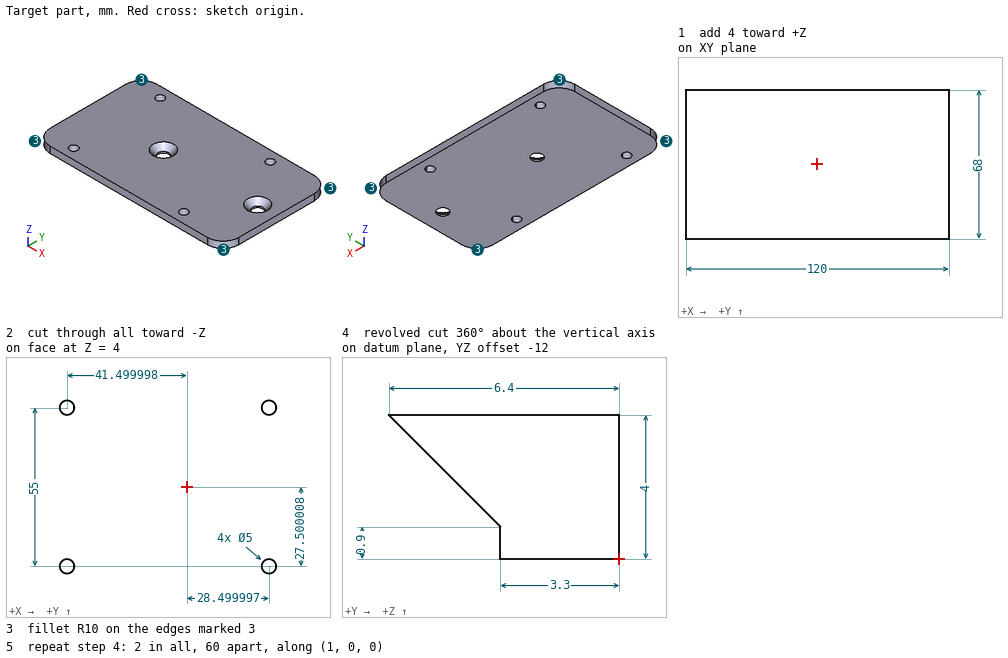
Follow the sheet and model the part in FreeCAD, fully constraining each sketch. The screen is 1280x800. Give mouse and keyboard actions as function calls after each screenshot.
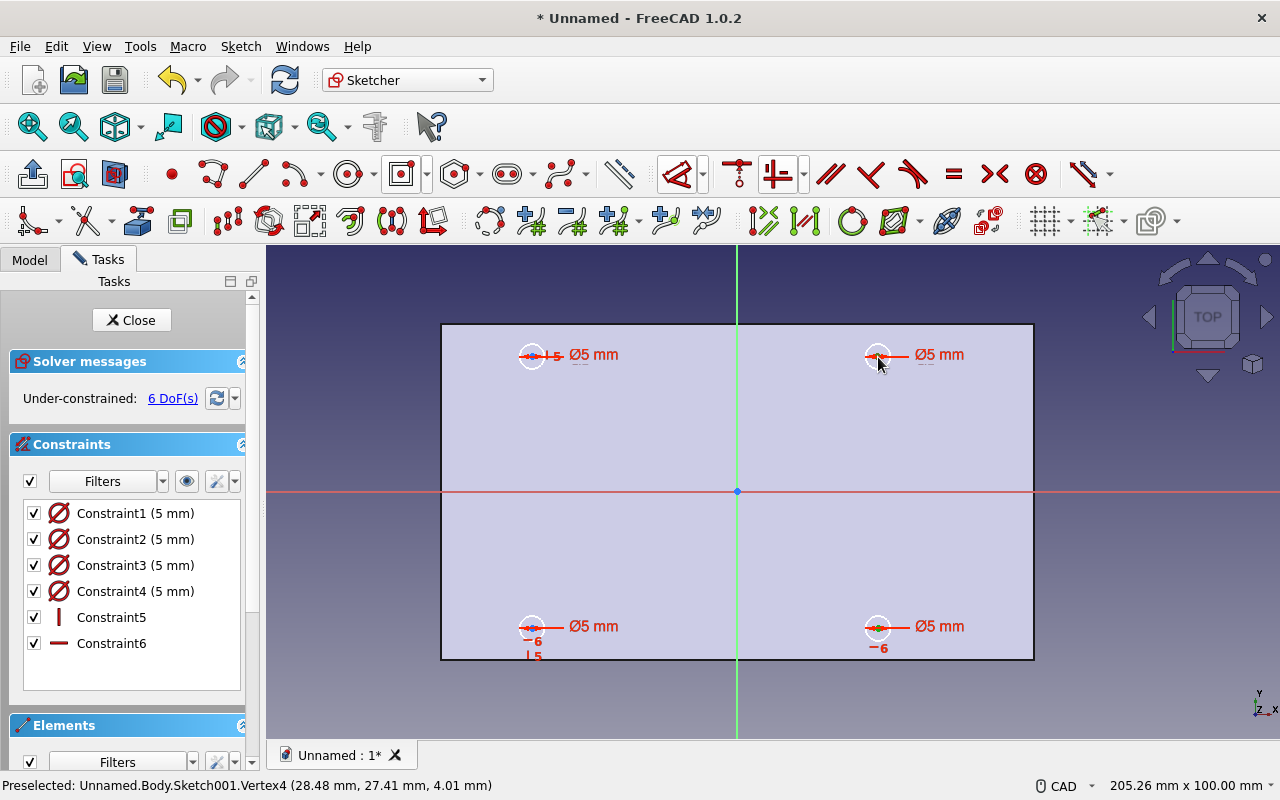
click(804, 174)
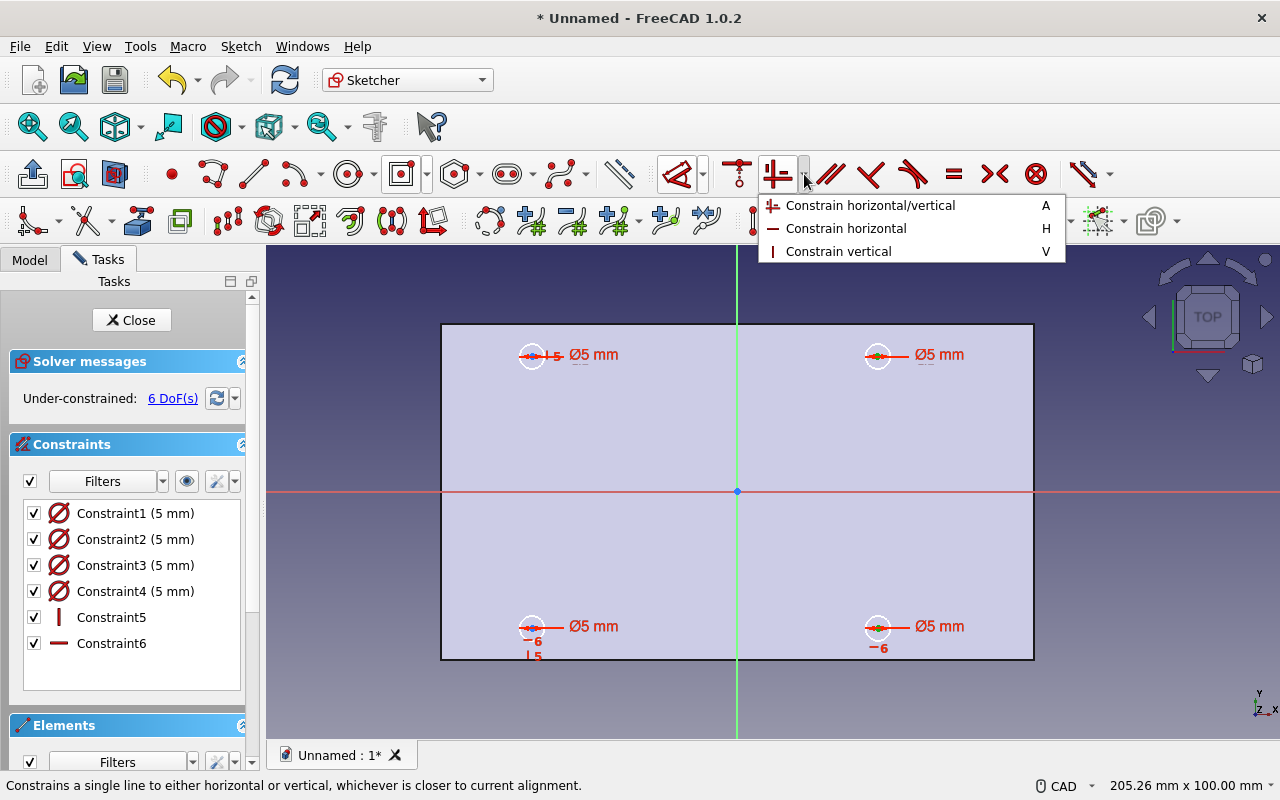
click(912, 252)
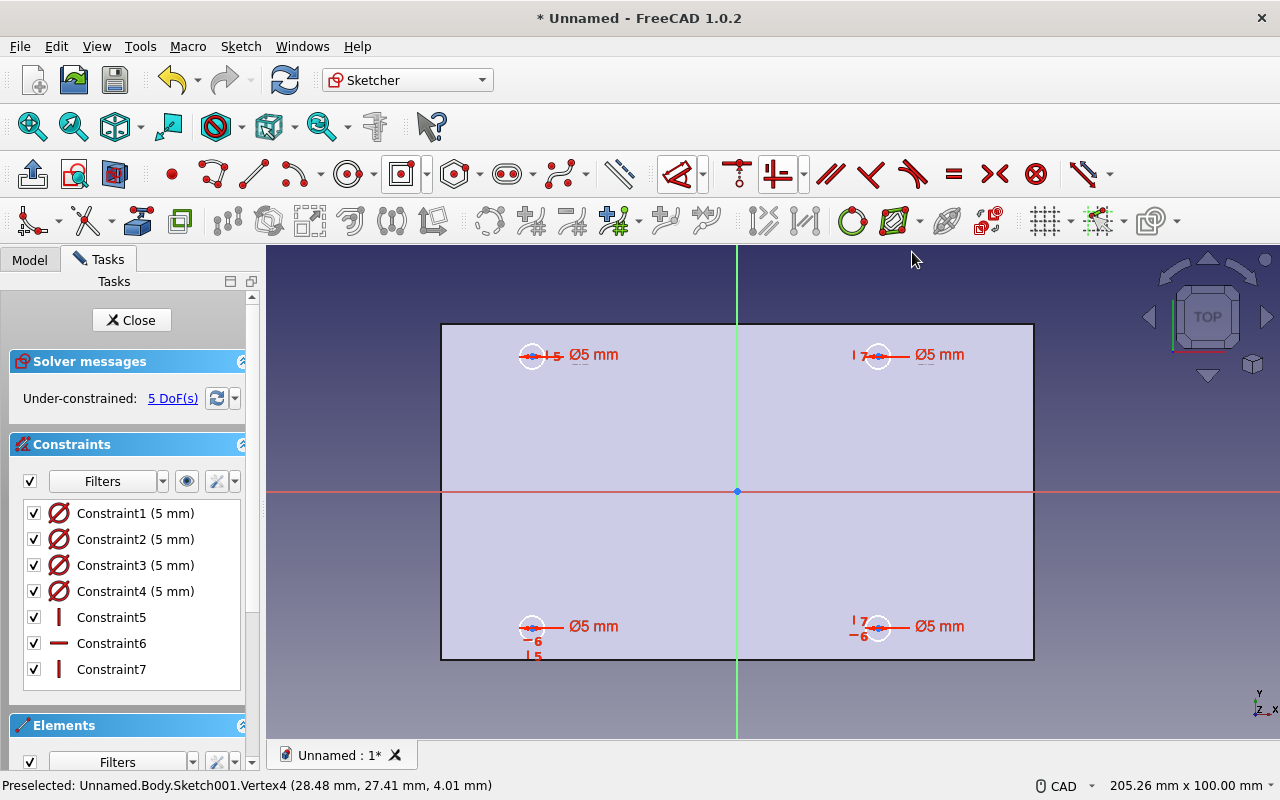
click(532, 357)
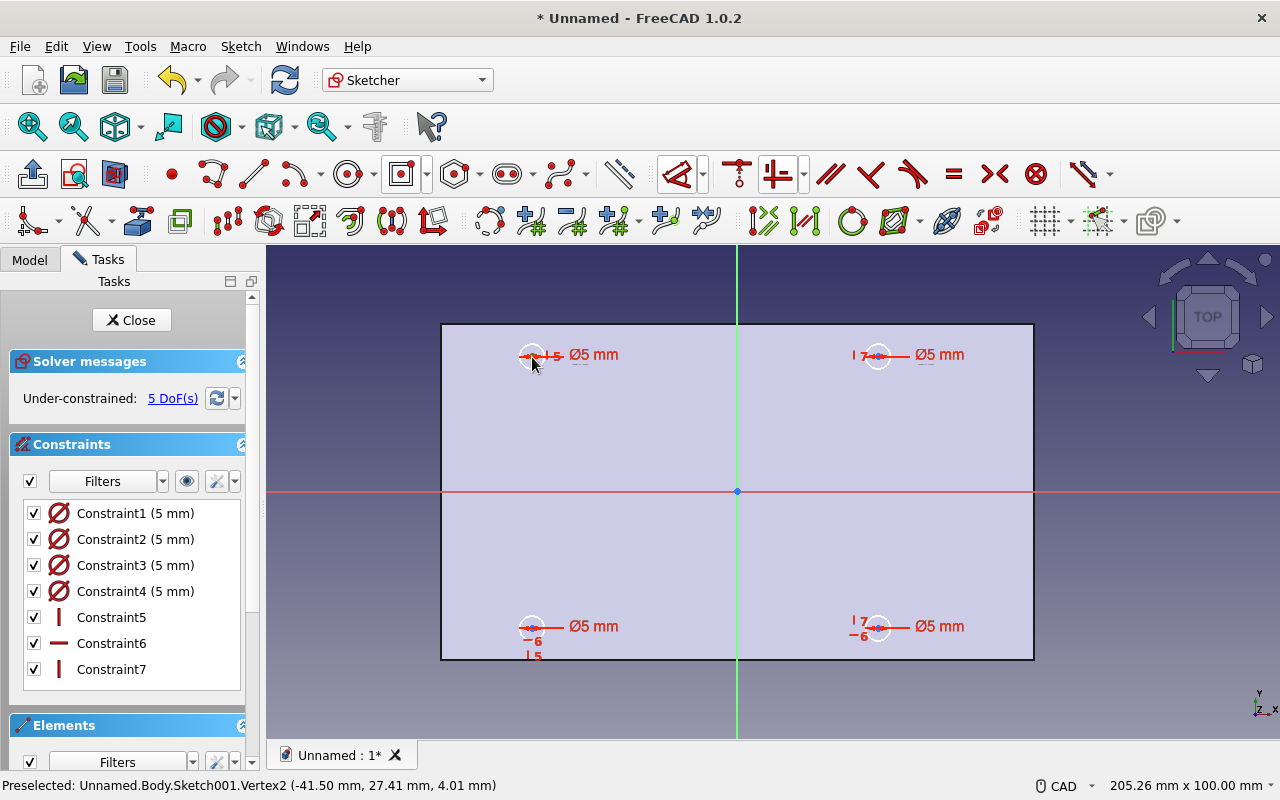
click(878, 357)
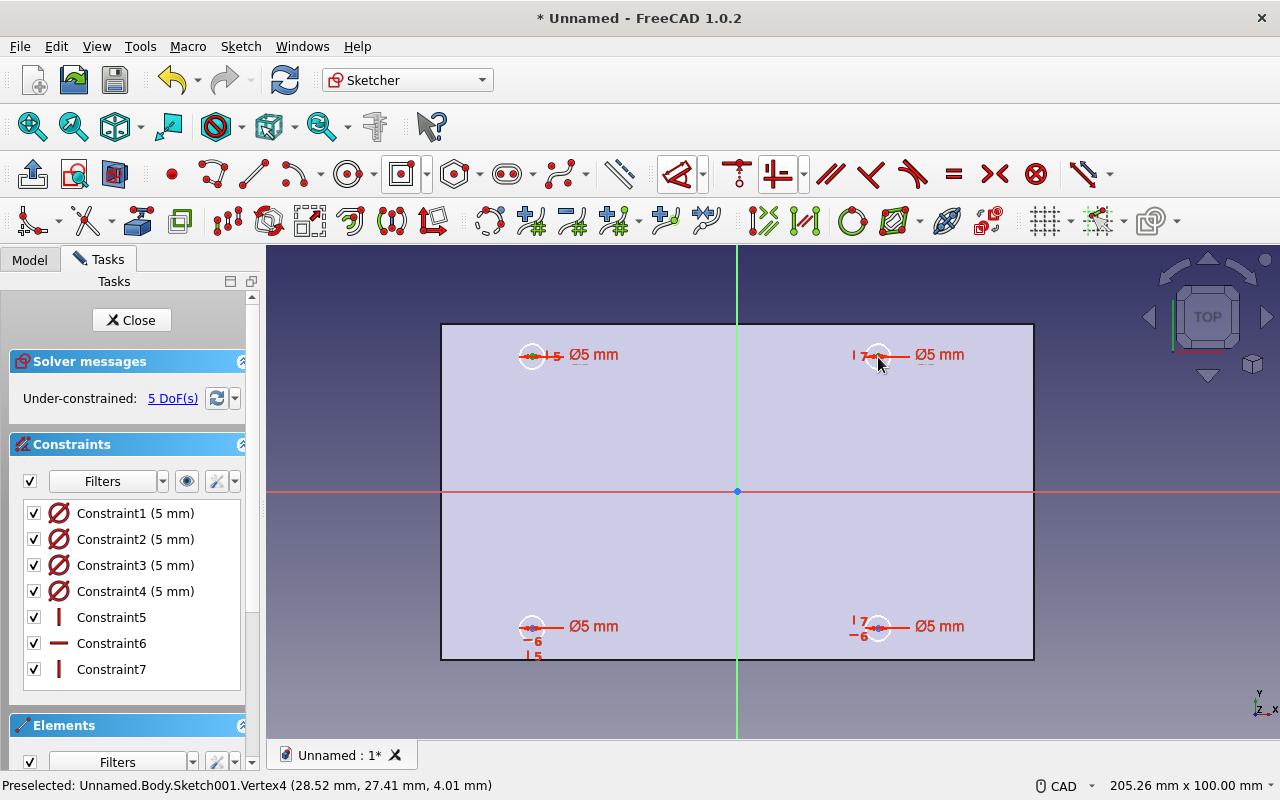
key(h)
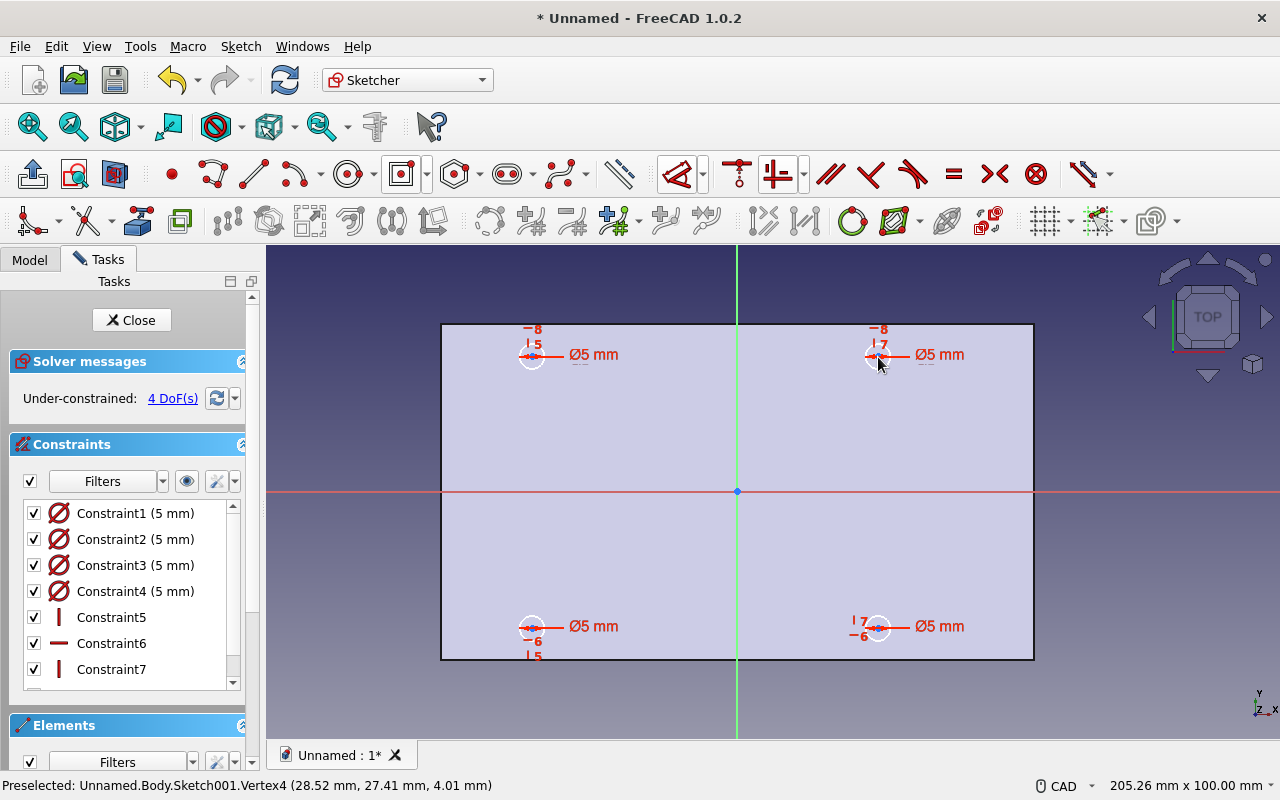
click(676, 174)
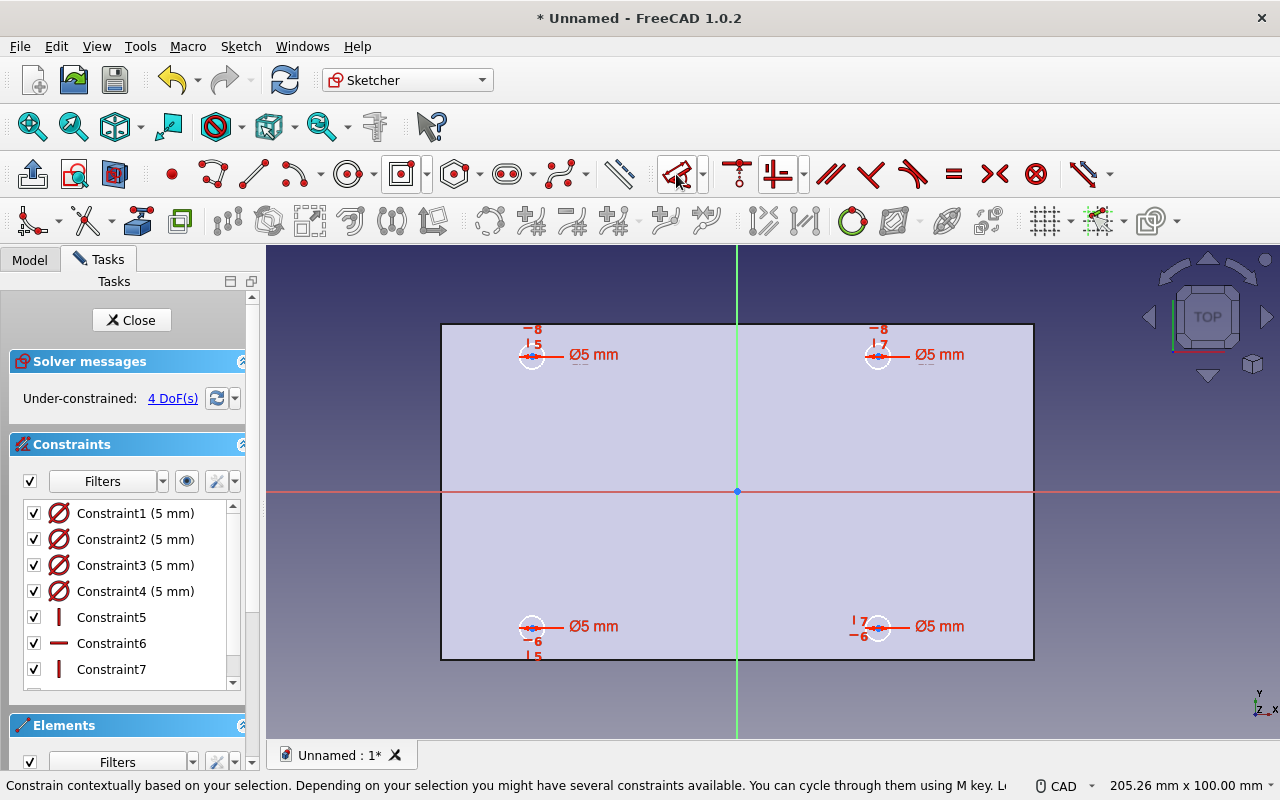
click(878, 628)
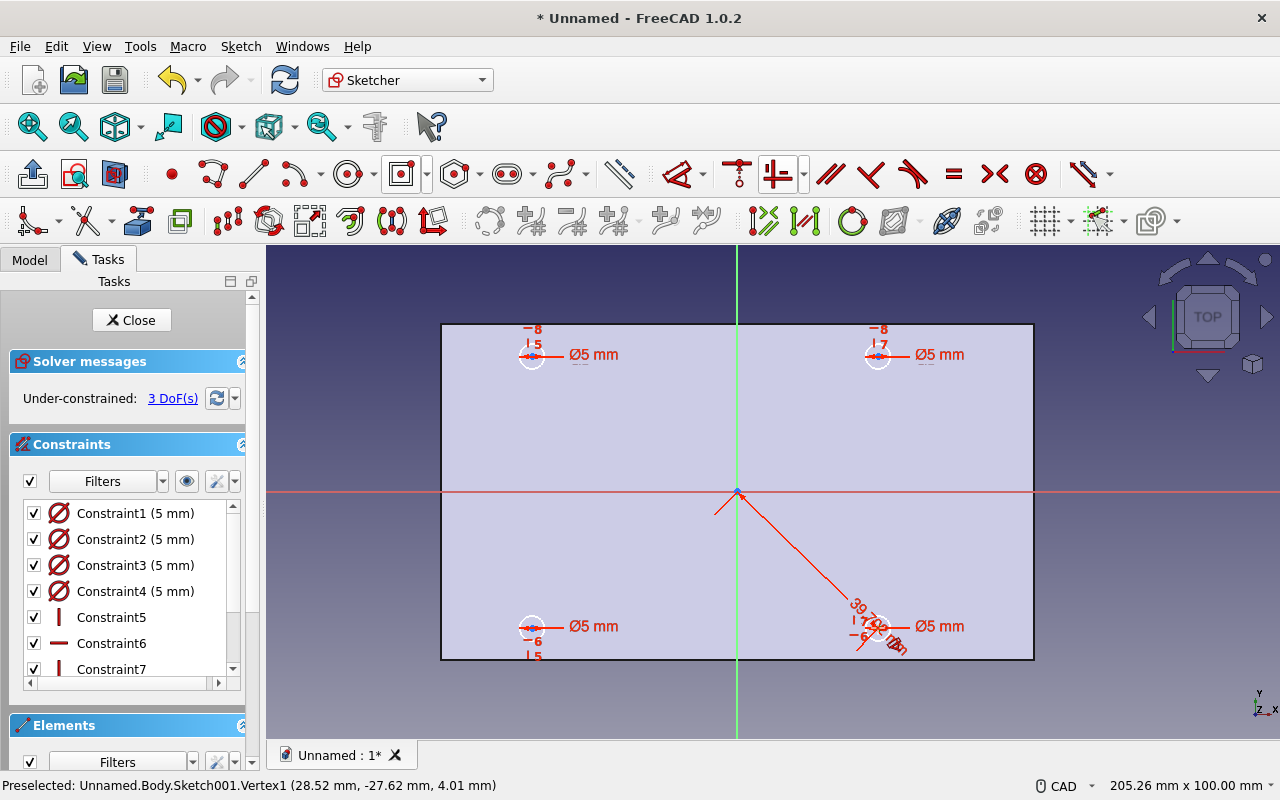
click(532, 357)
click(912, 430)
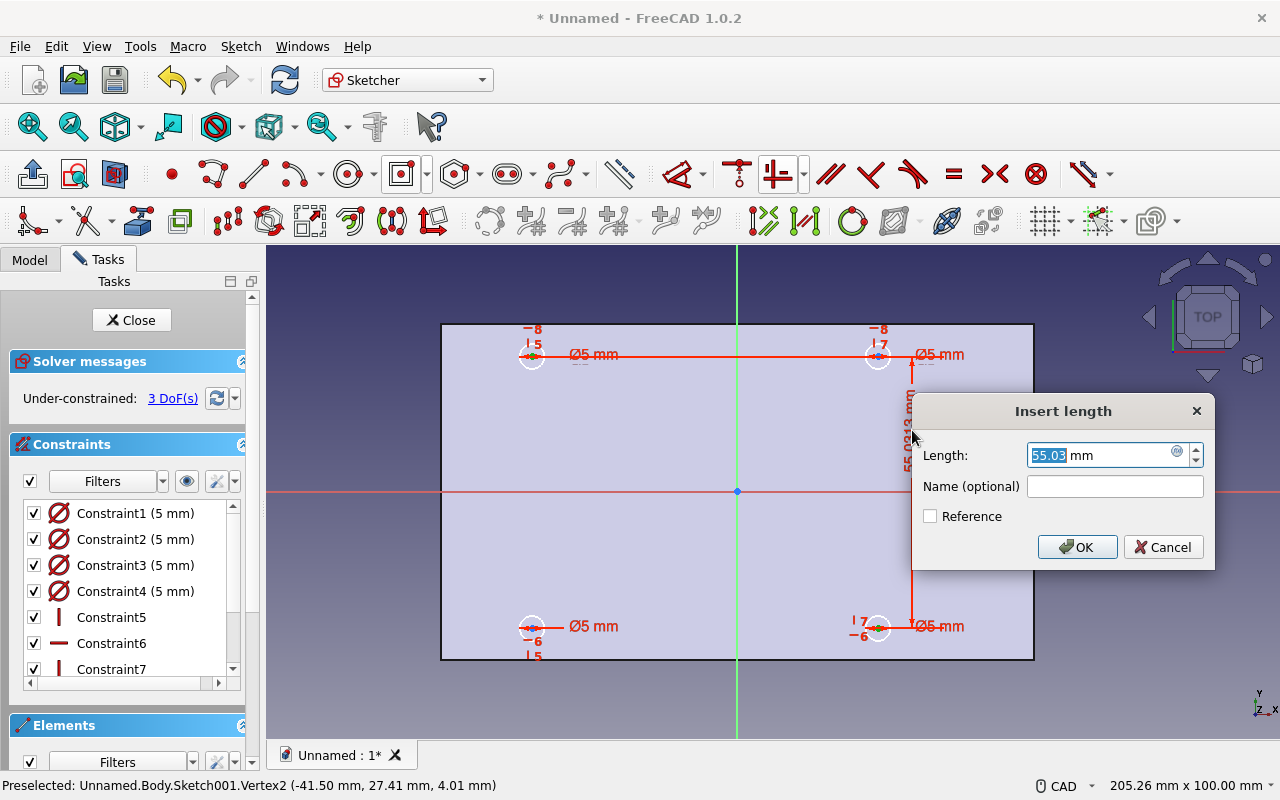
text(55)
key(Return)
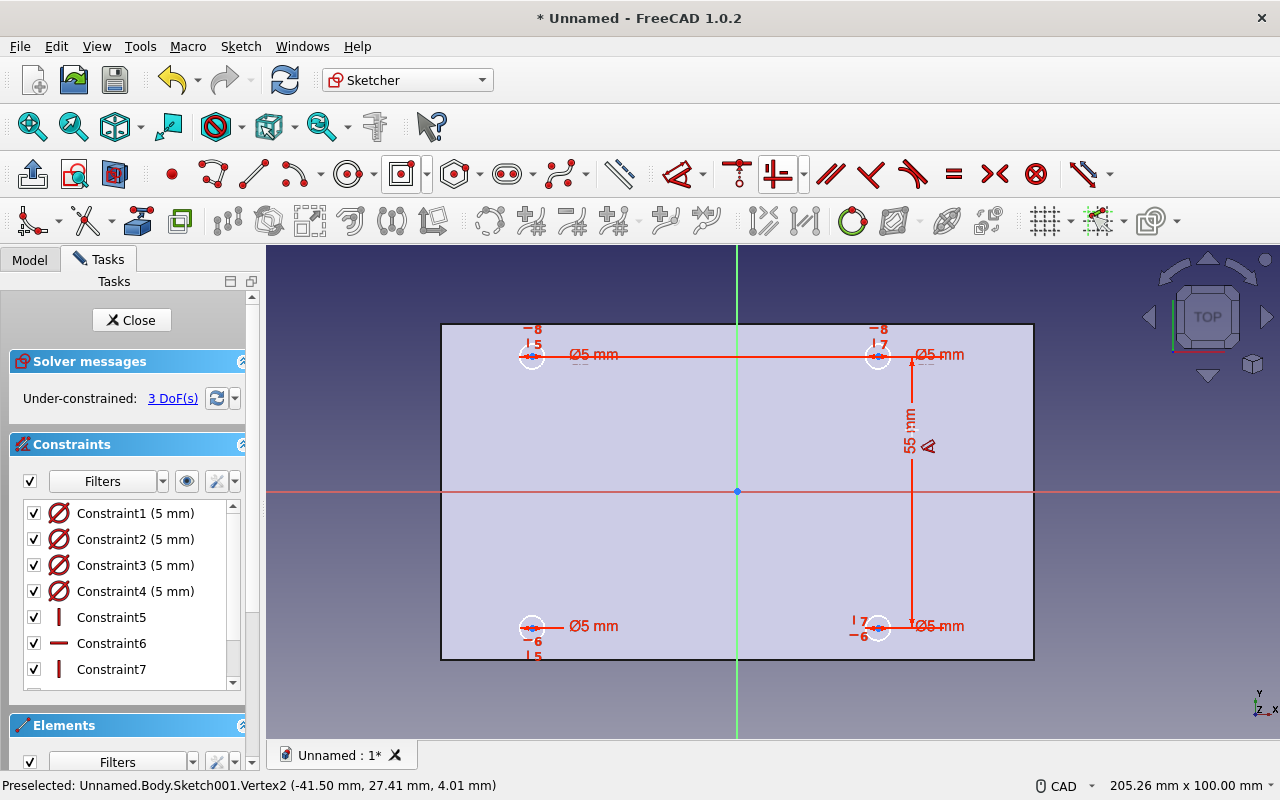
click(878, 628)
click(808, 662)